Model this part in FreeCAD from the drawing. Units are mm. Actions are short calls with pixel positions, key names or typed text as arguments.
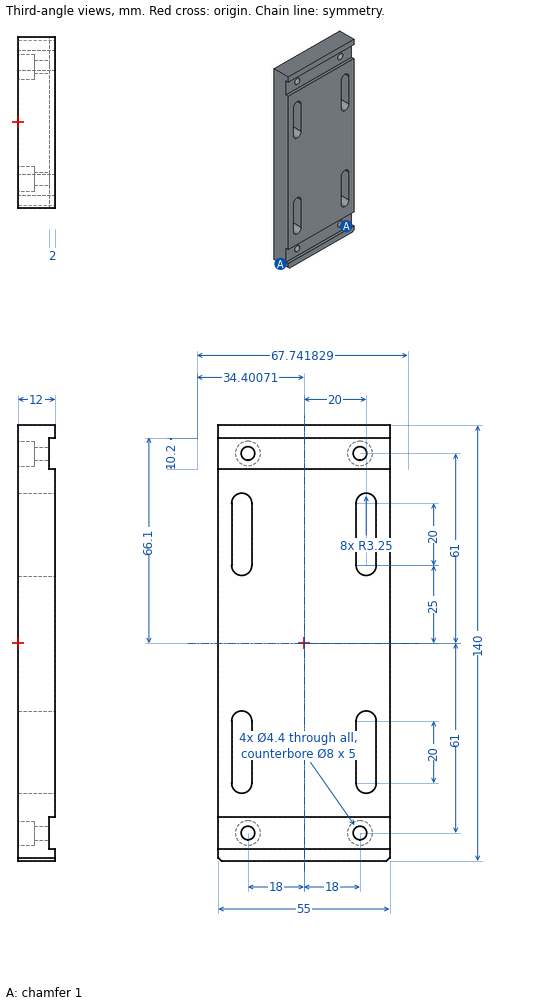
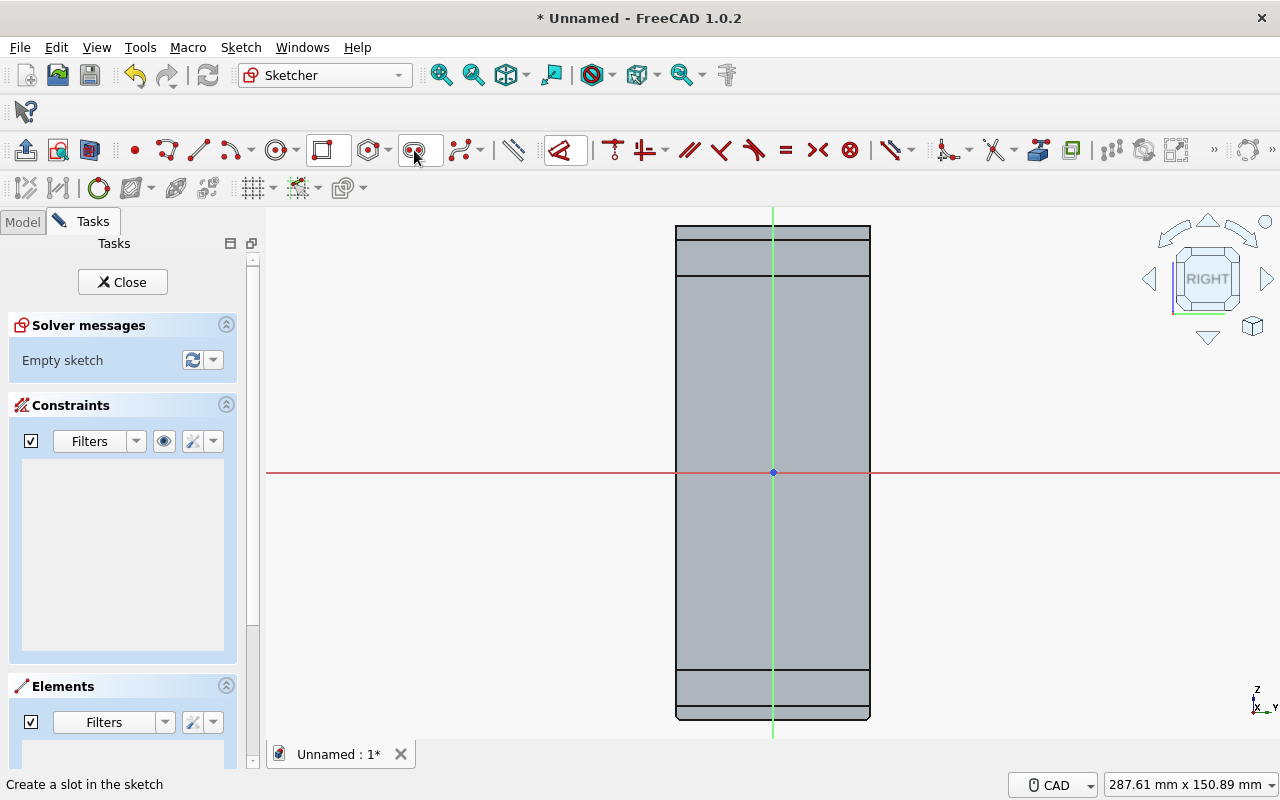
scroll(844, 385, up, 4)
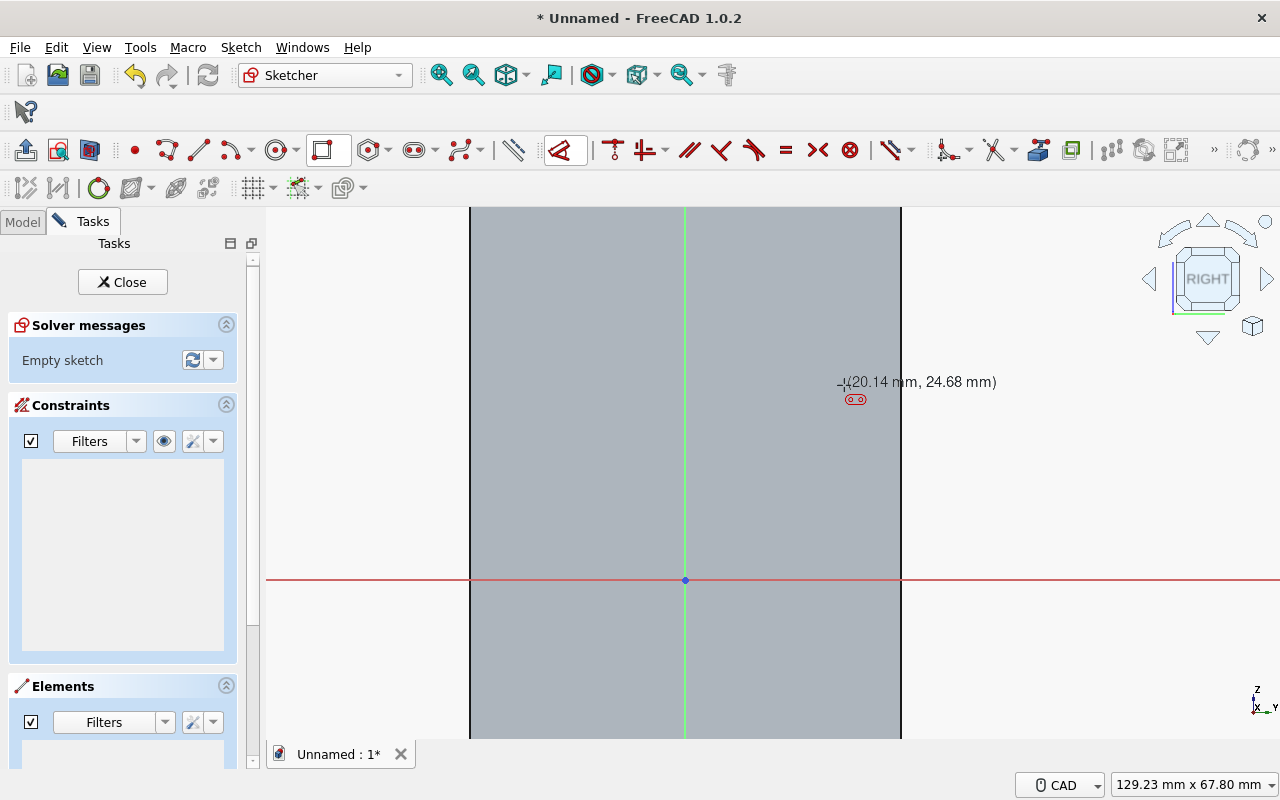
click(842, 384)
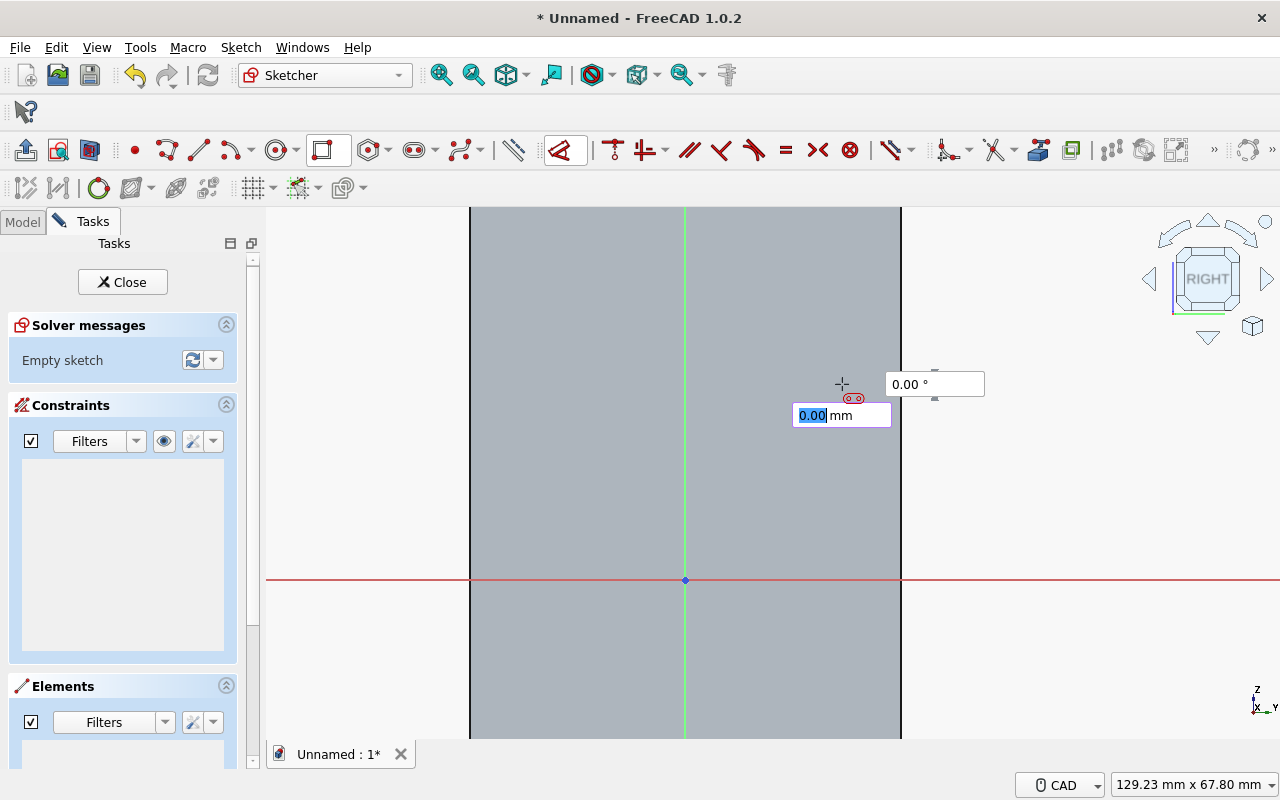
scroll(720, 385, down, 4)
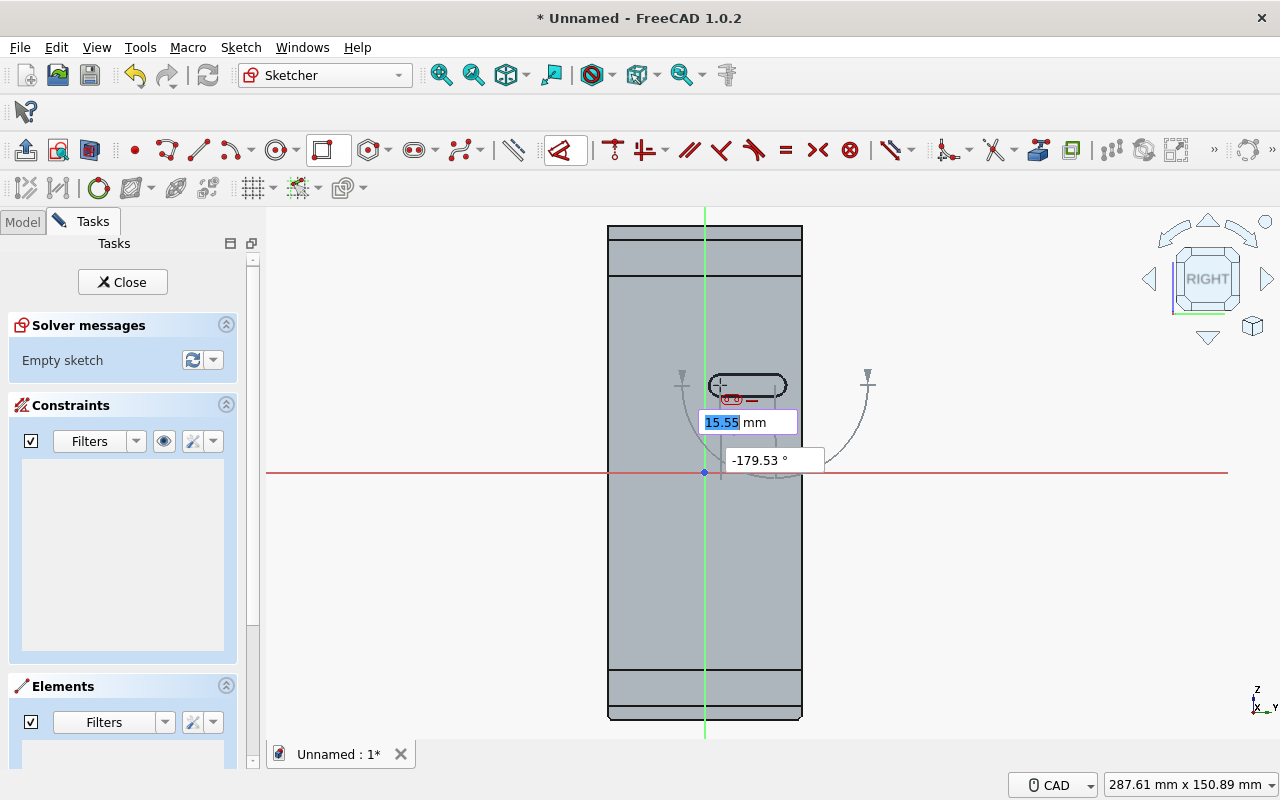
click(775, 314)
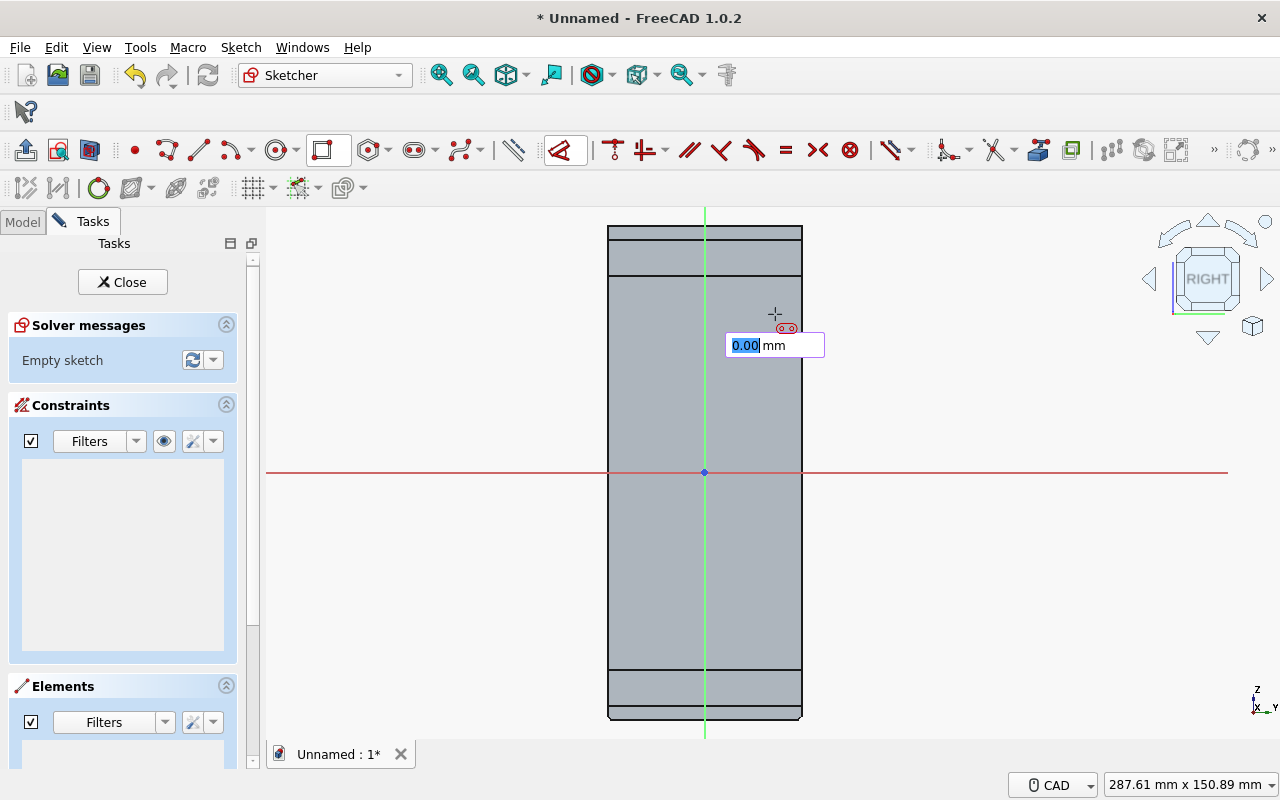
scroll(787, 350, up, 2)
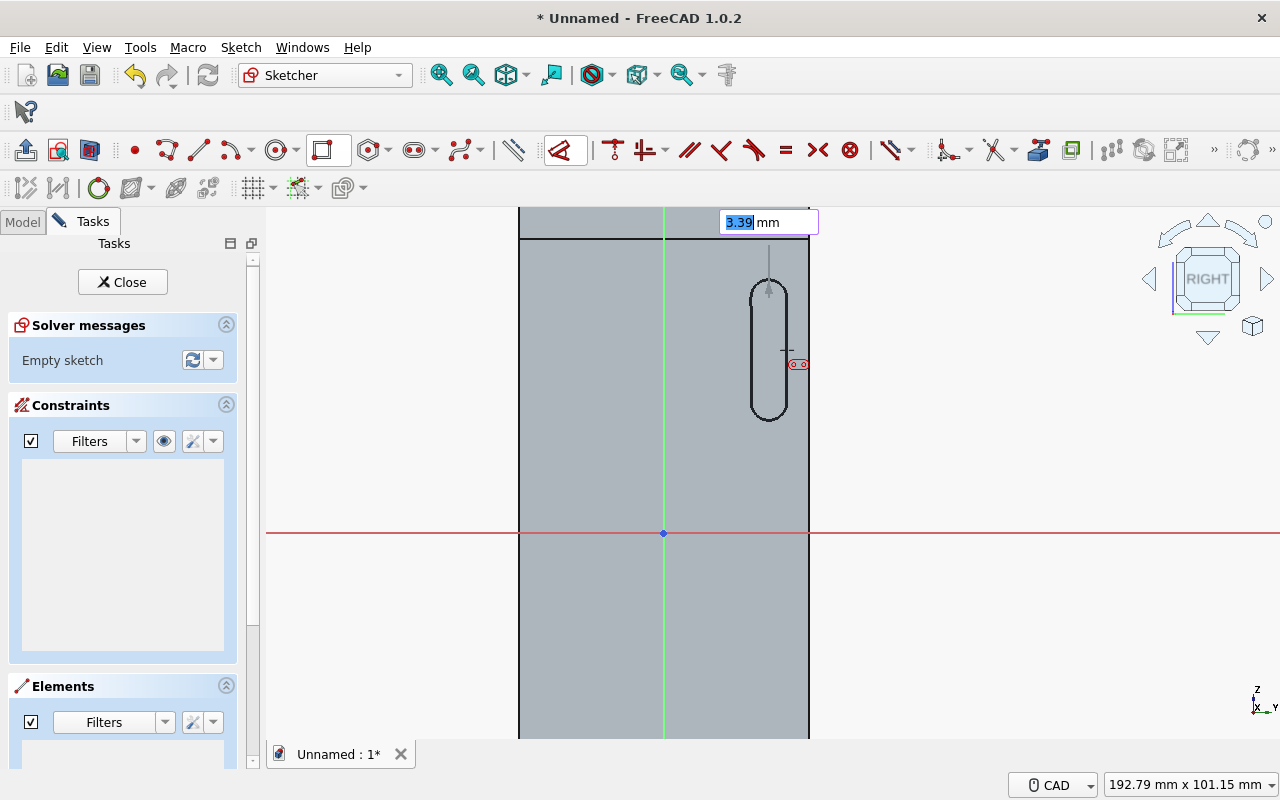
click(786, 349)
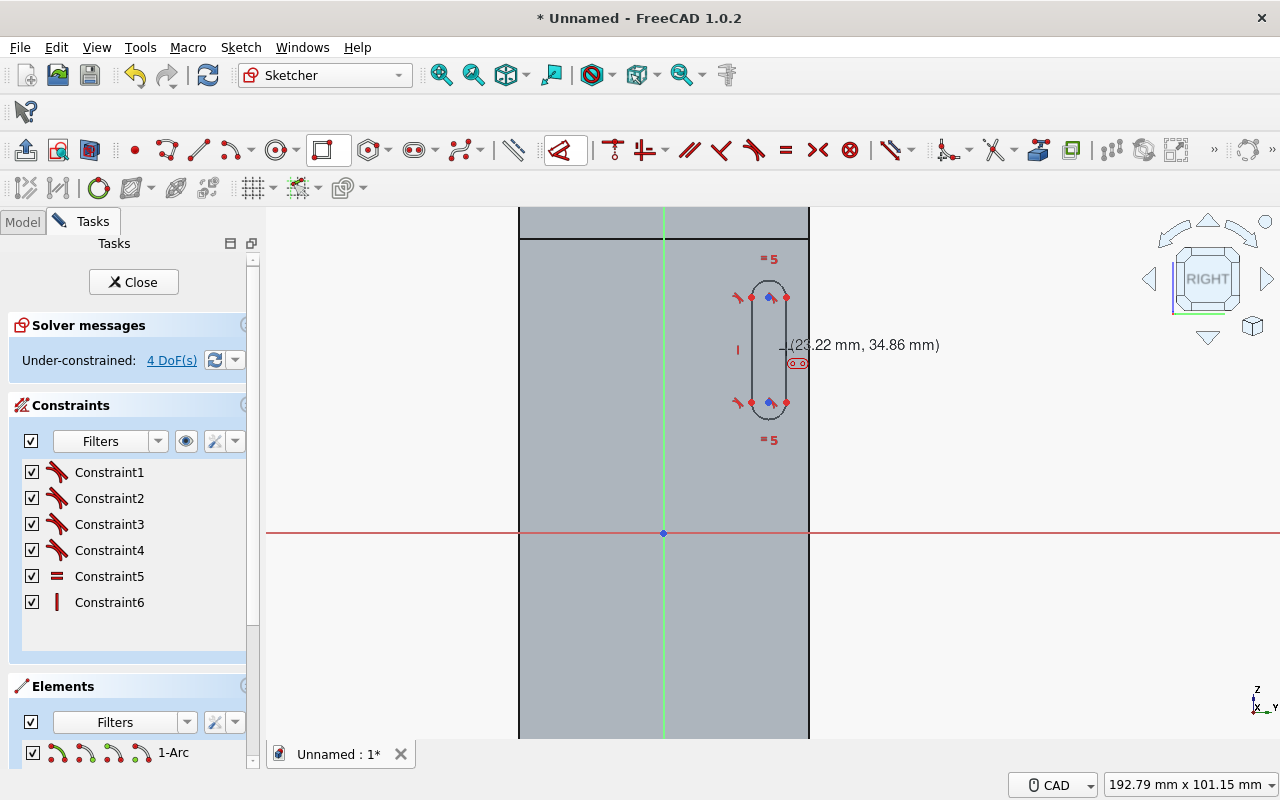
scroll(559, 402, up, 2)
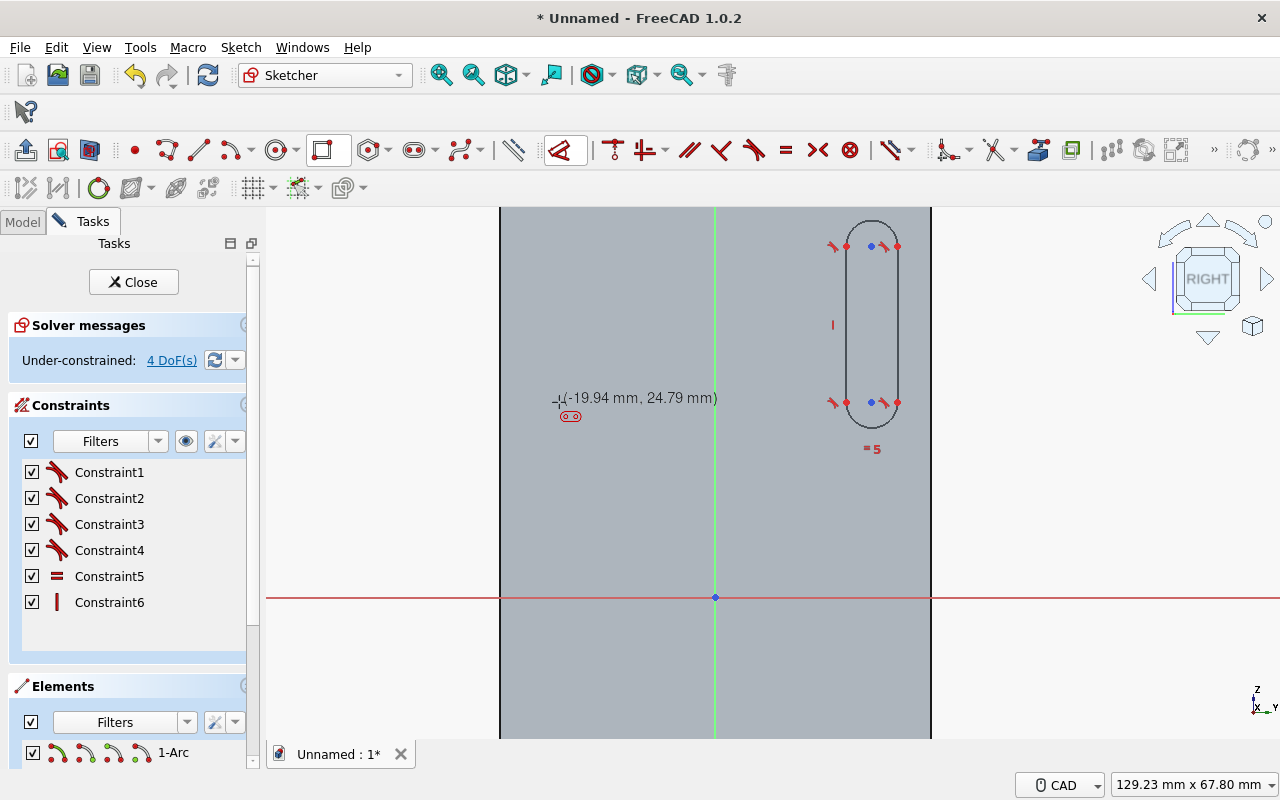
click(558, 402)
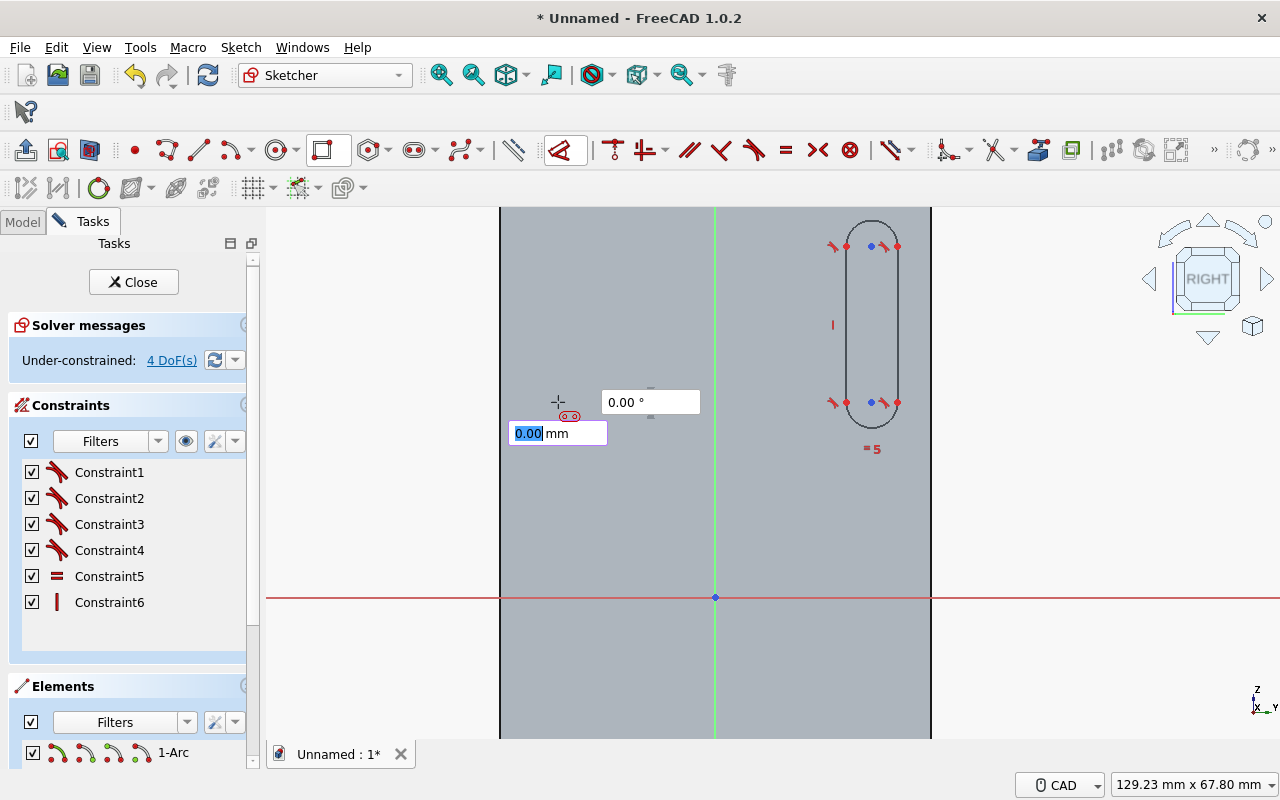
click(558, 245)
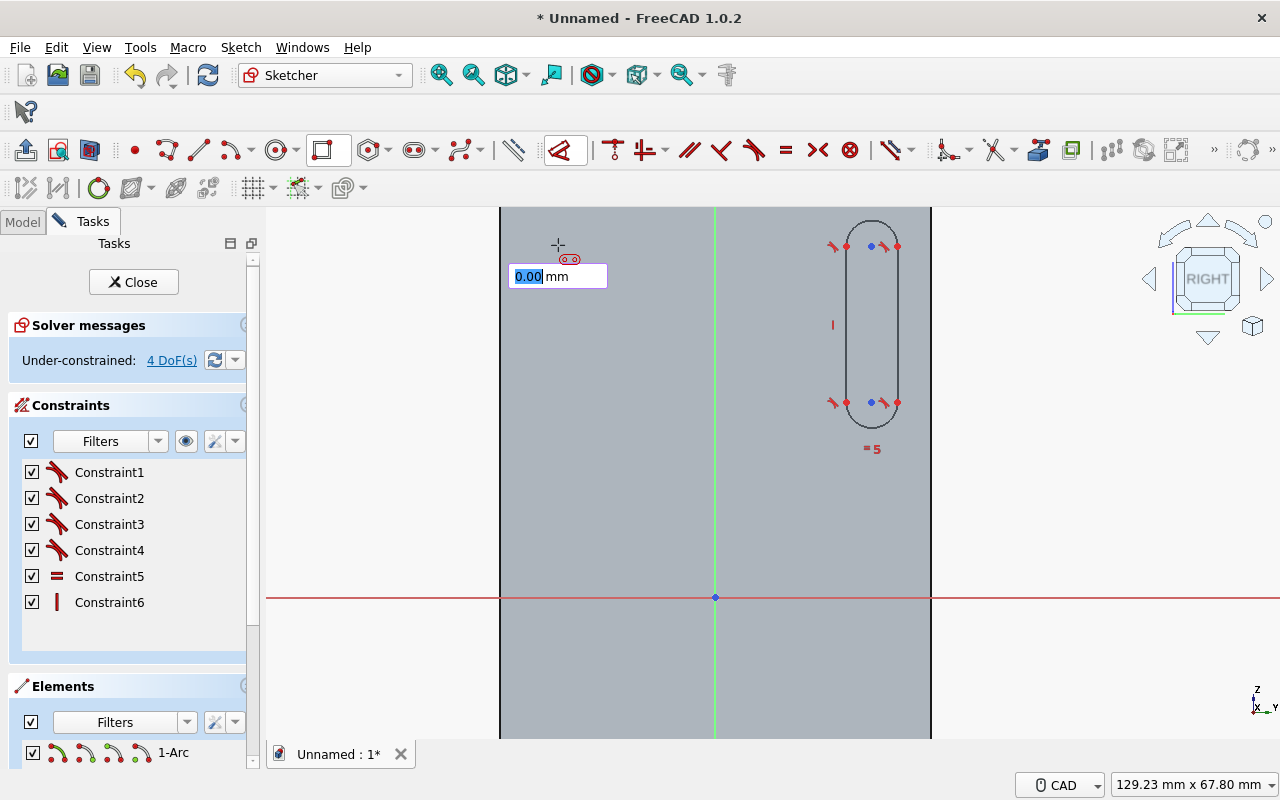
click(533, 323)